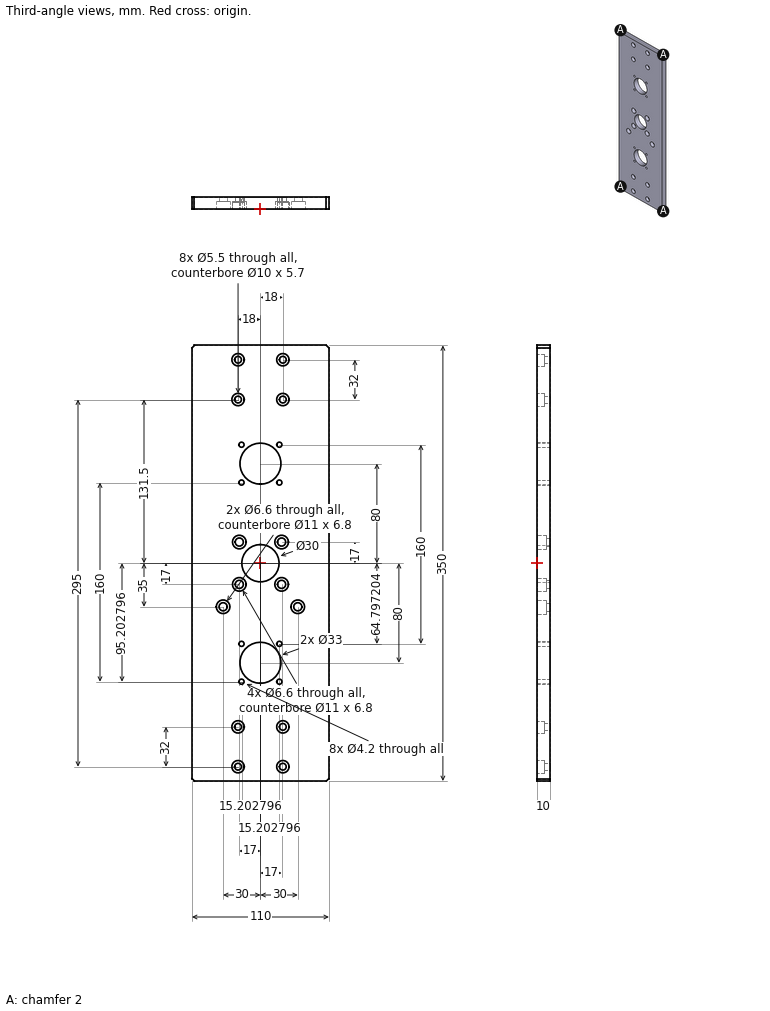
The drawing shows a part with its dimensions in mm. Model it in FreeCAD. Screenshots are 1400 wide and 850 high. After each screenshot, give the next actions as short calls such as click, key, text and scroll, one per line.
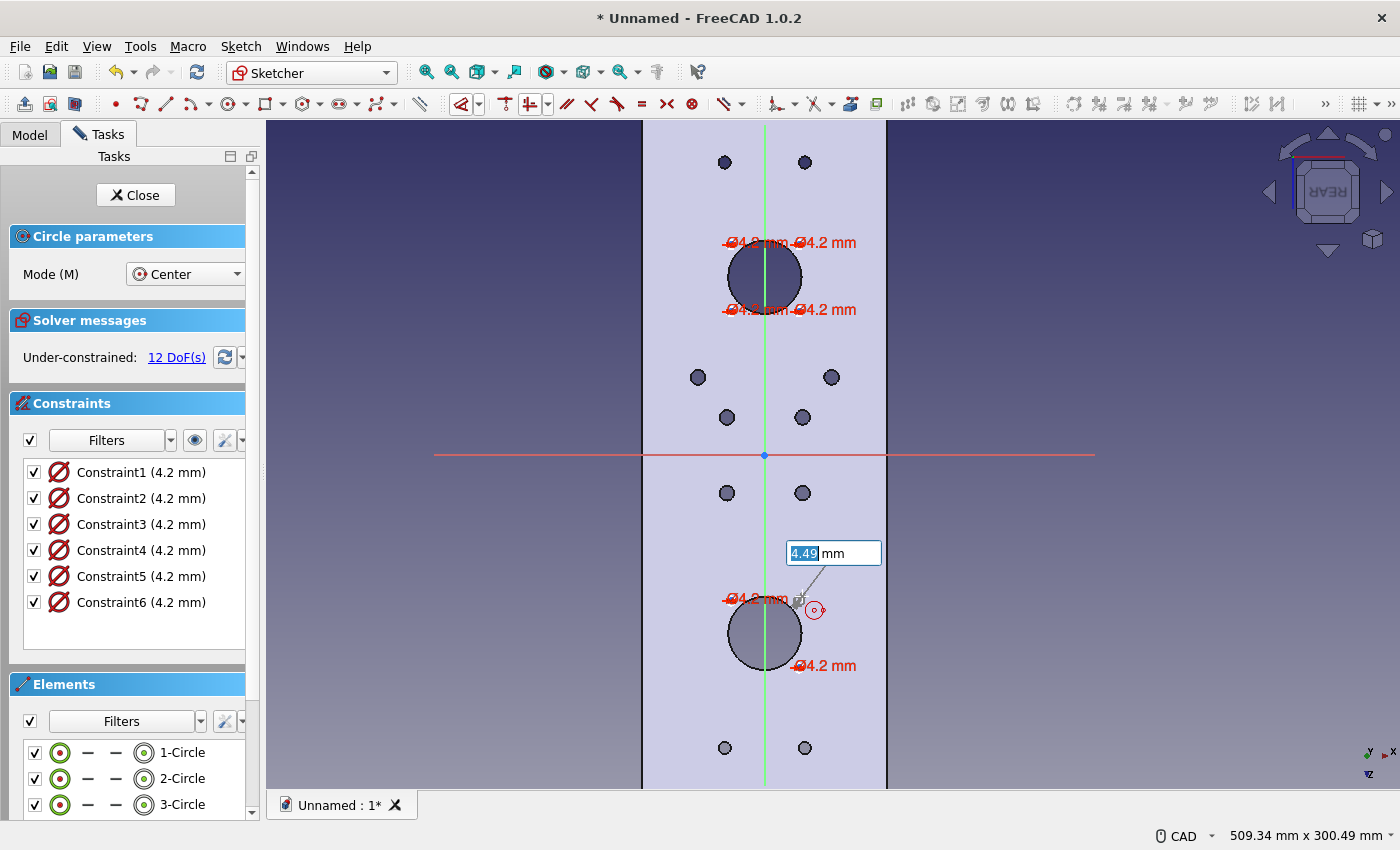
text(4.2)
key(Return)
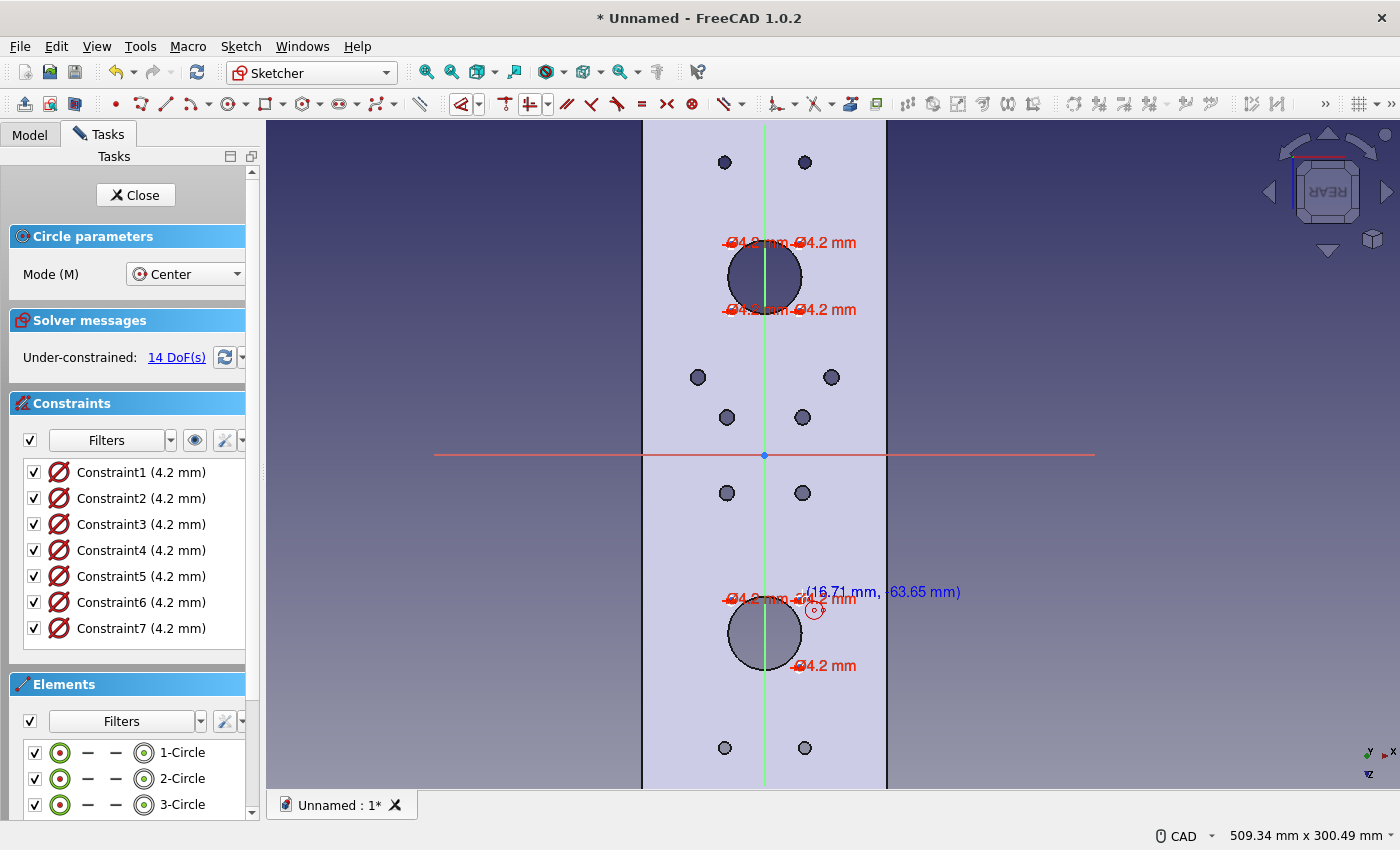
scroll(731, 667, up, 8)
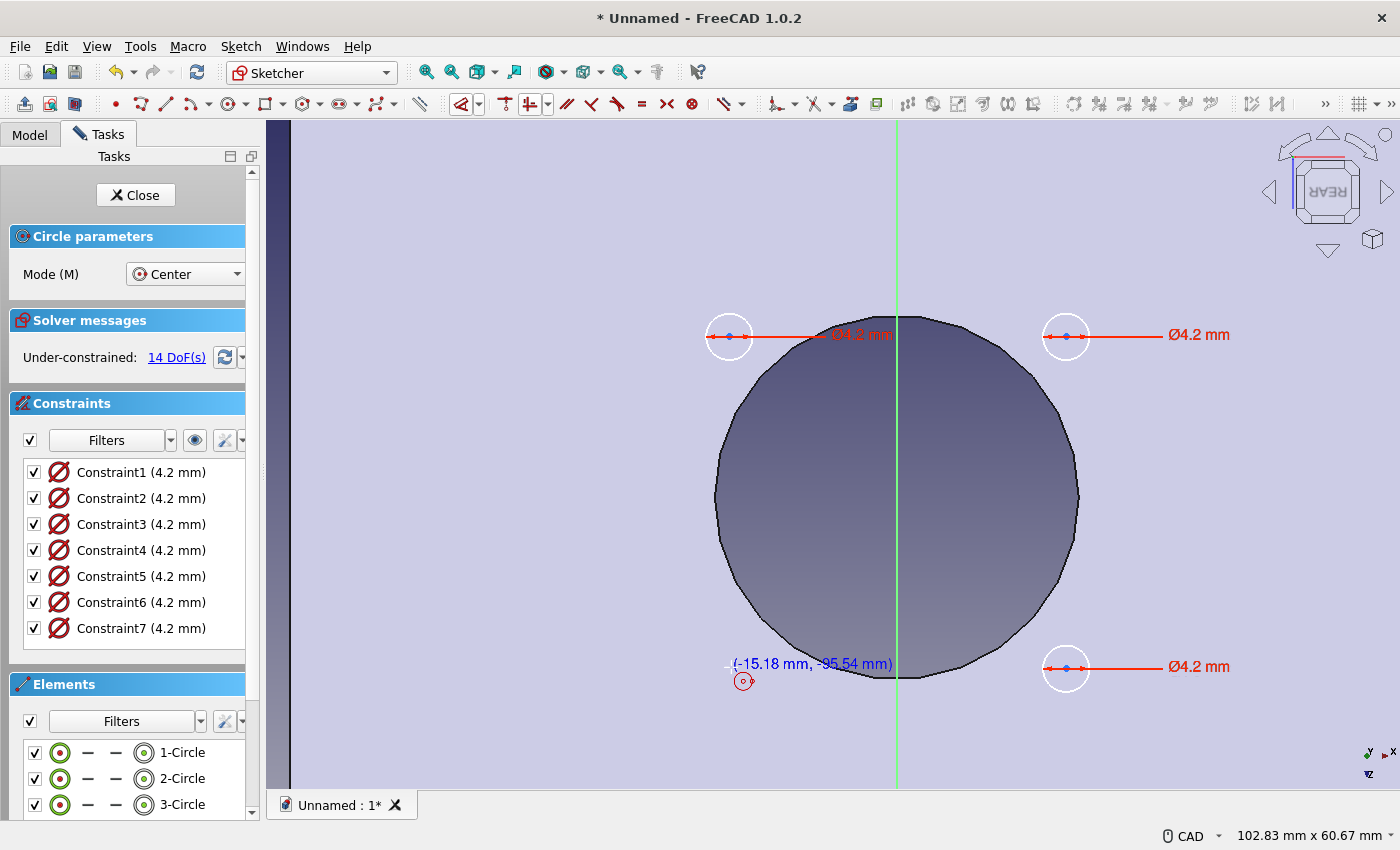
scroll(731, 667, down, 8)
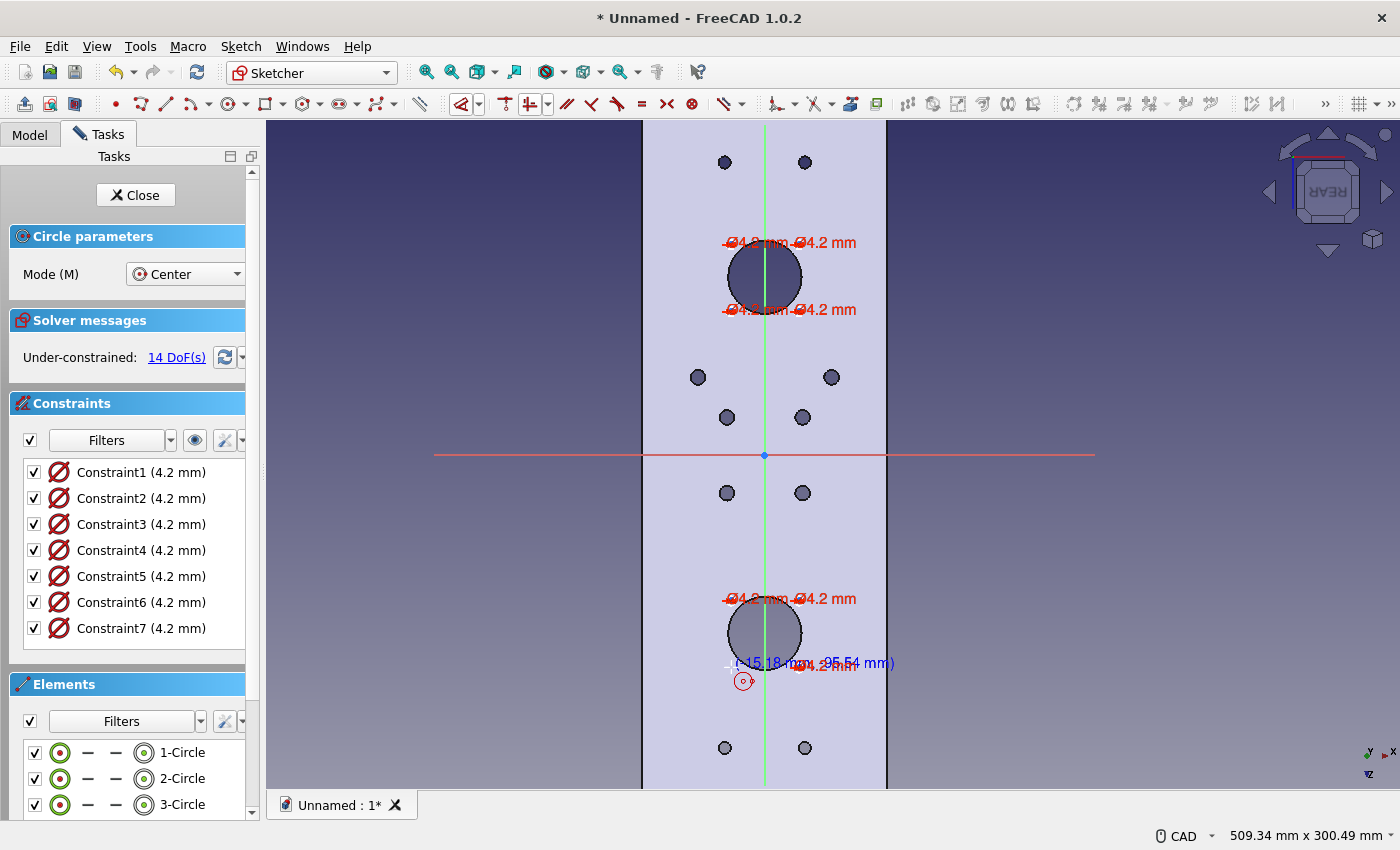
click(731, 667)
move(734, 664)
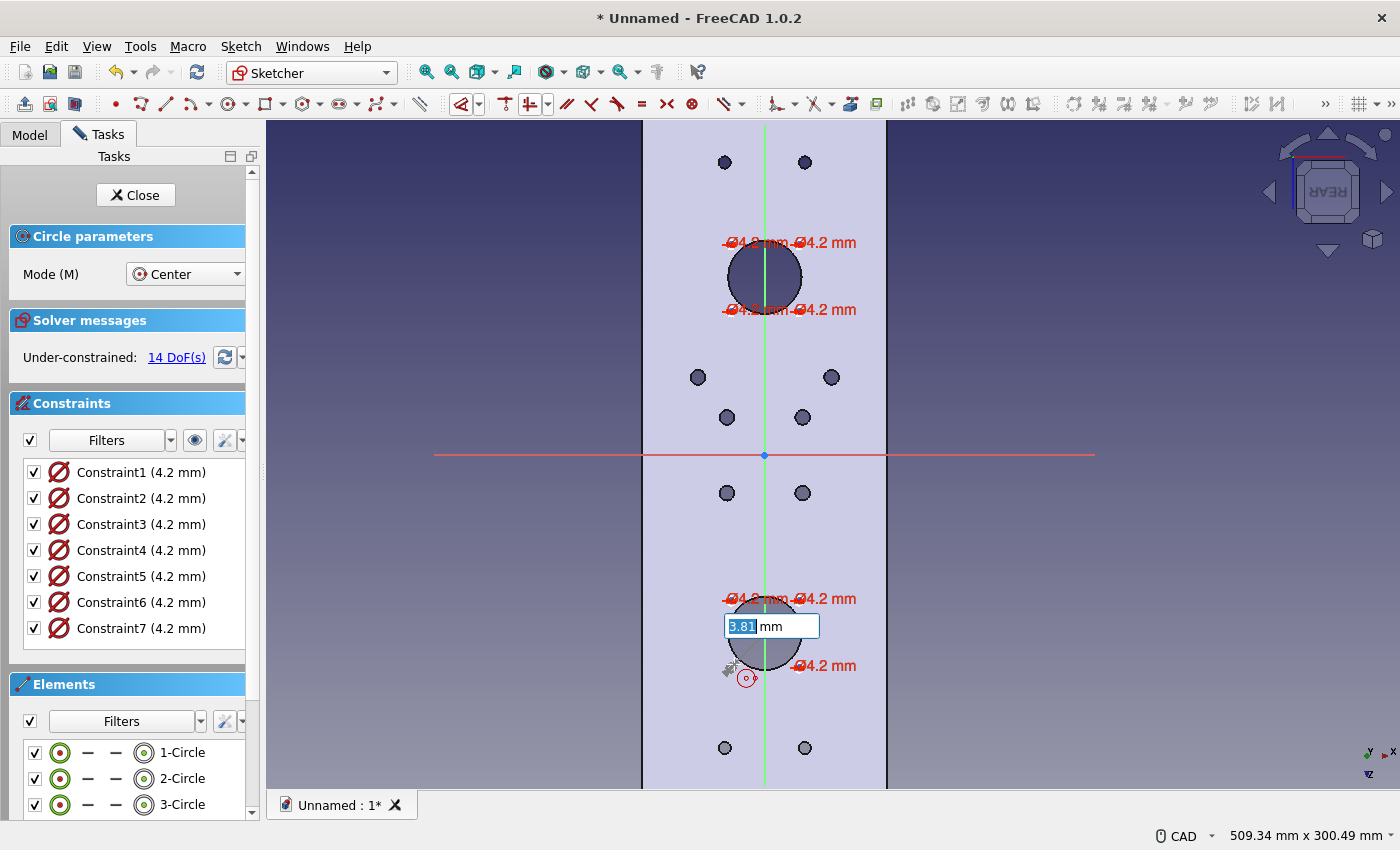
text(4.2)
key(Return)
key(Escape)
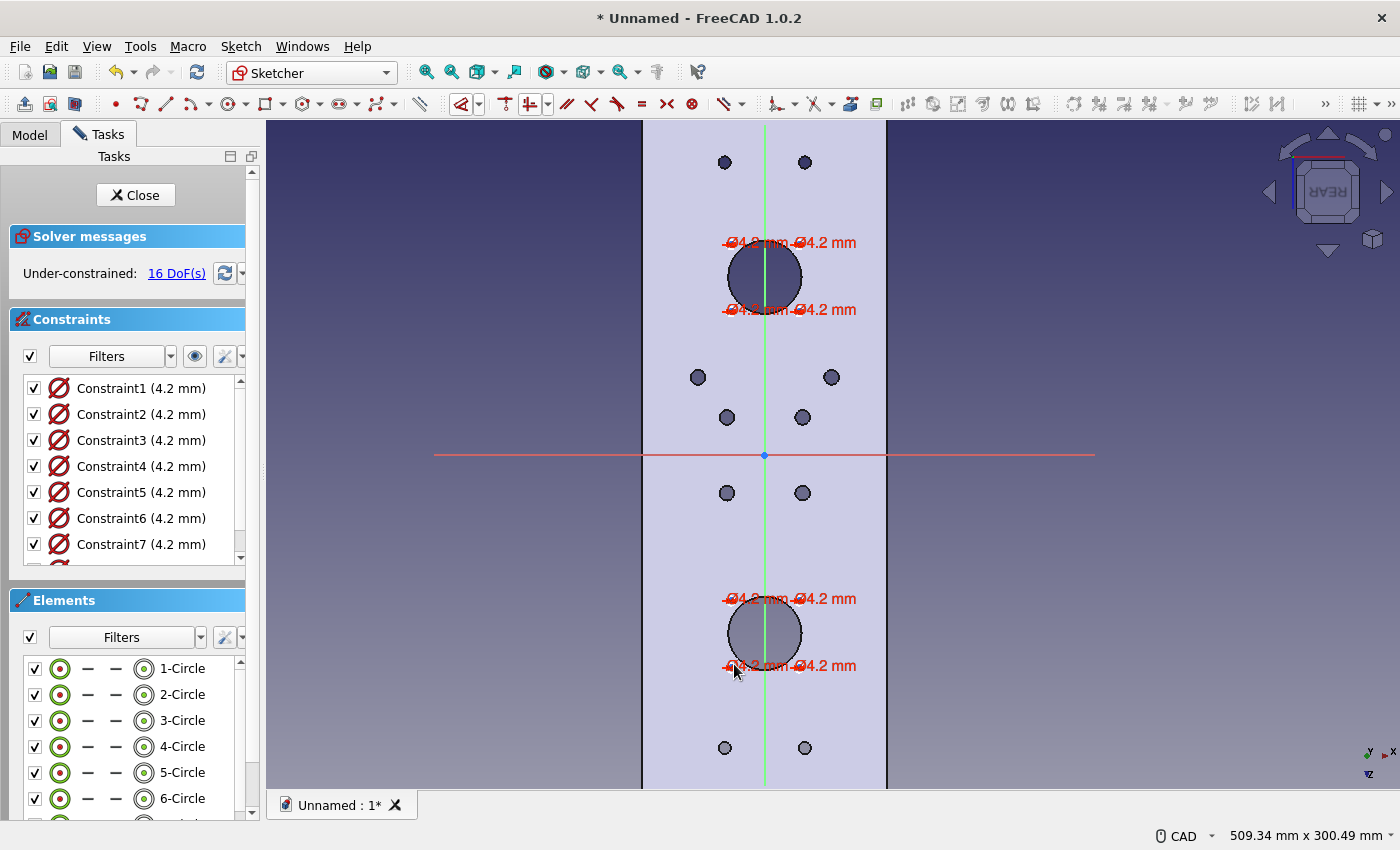
click(731, 245)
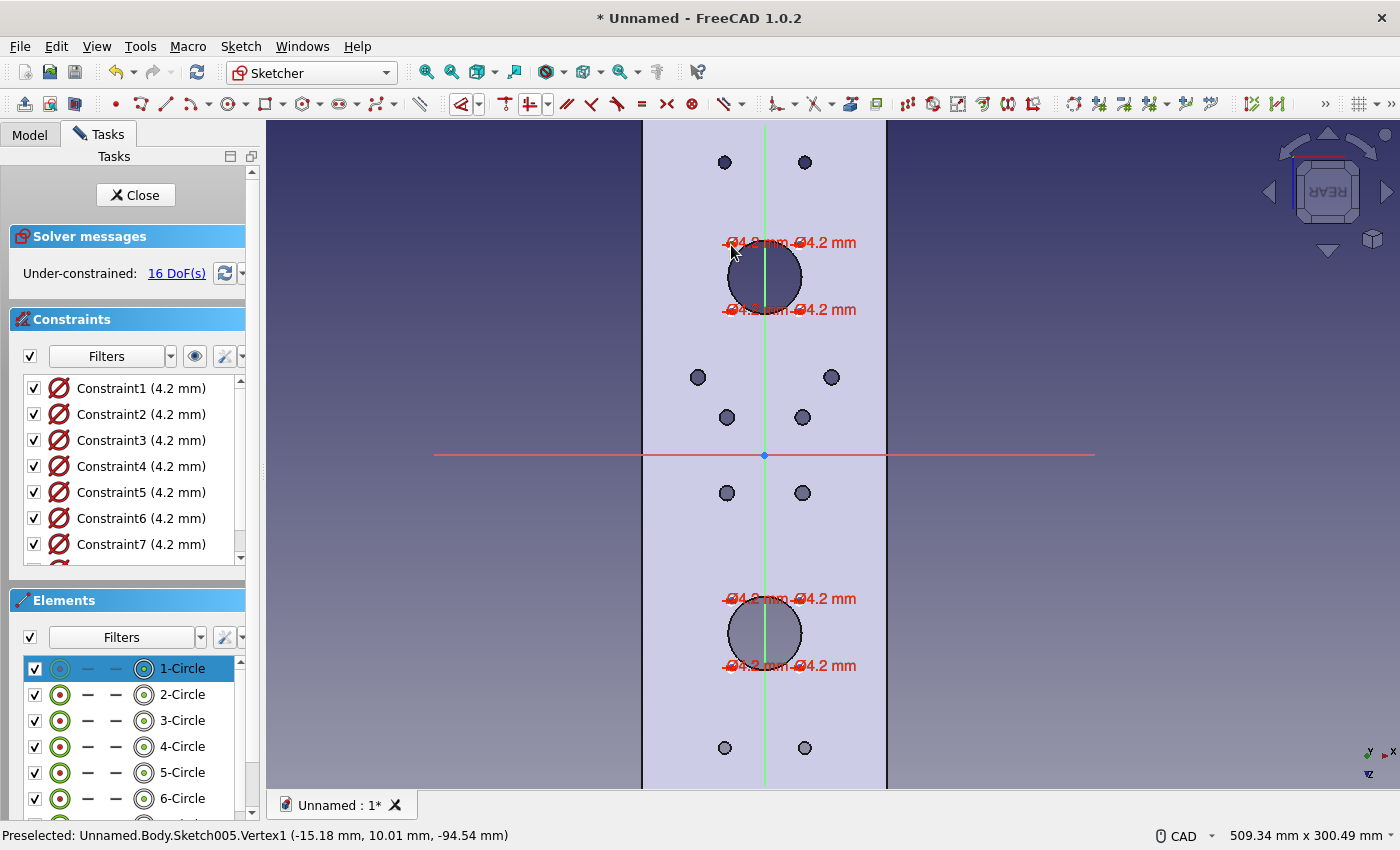
click(731, 312)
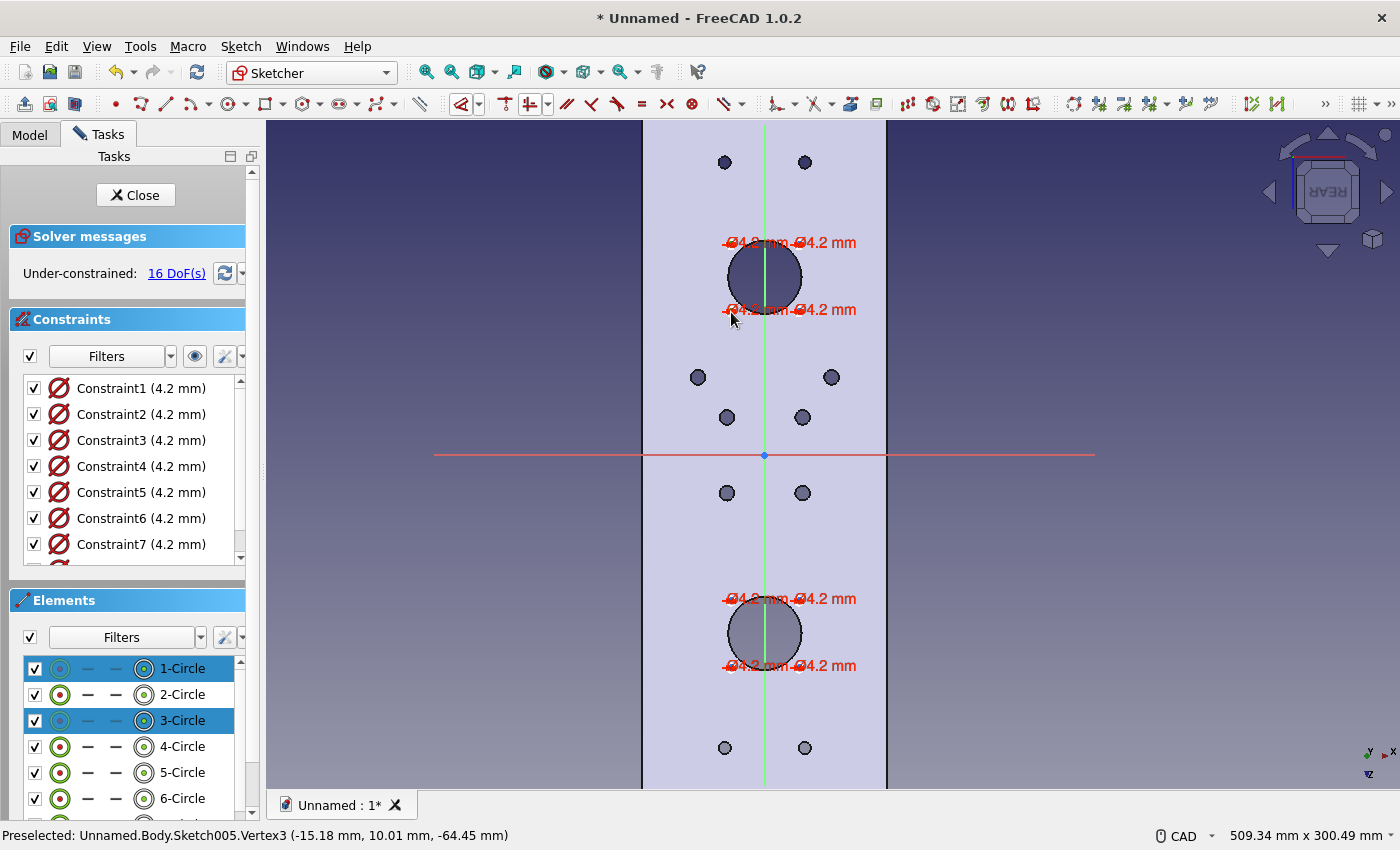
key(v)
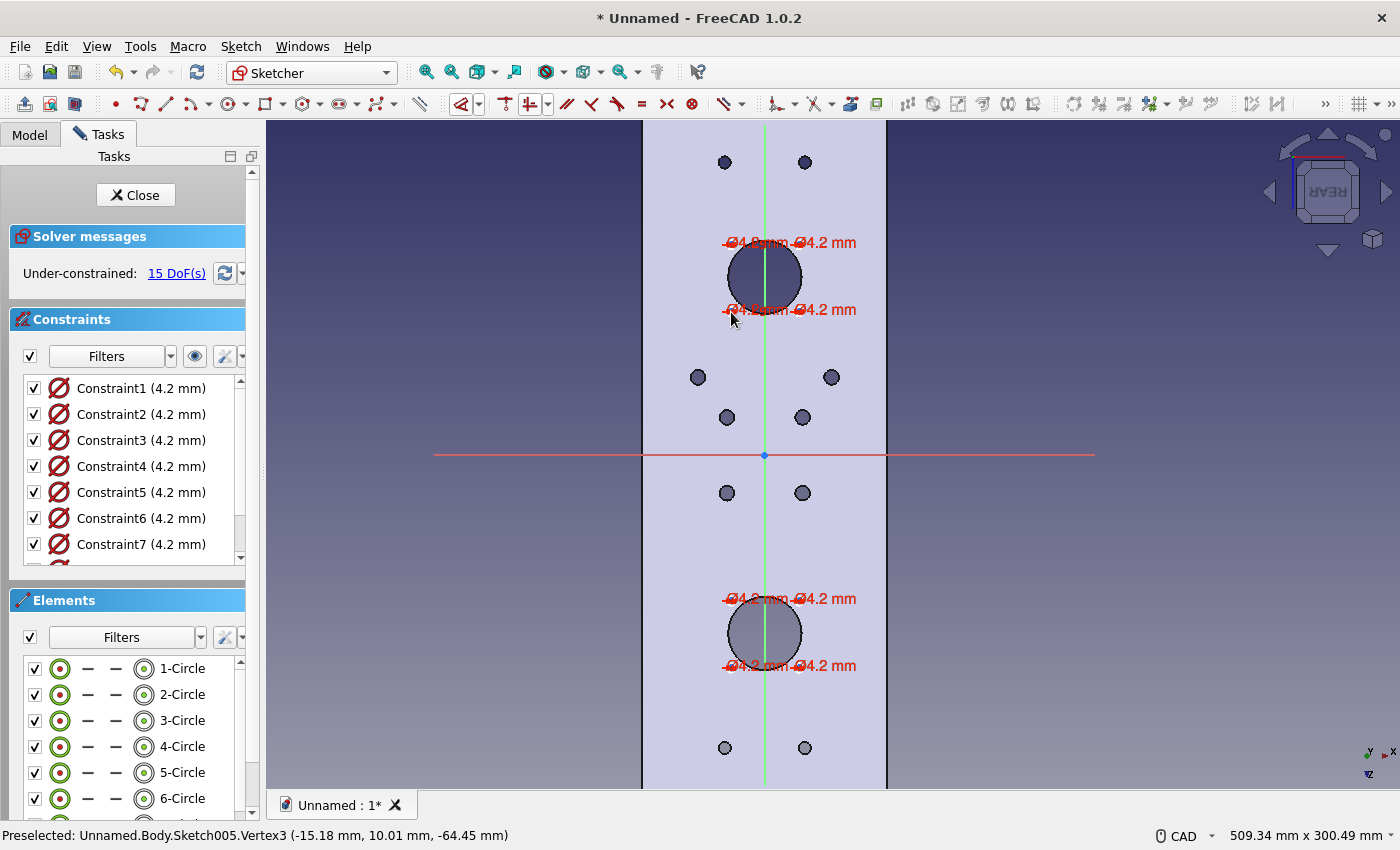
click(799, 312)